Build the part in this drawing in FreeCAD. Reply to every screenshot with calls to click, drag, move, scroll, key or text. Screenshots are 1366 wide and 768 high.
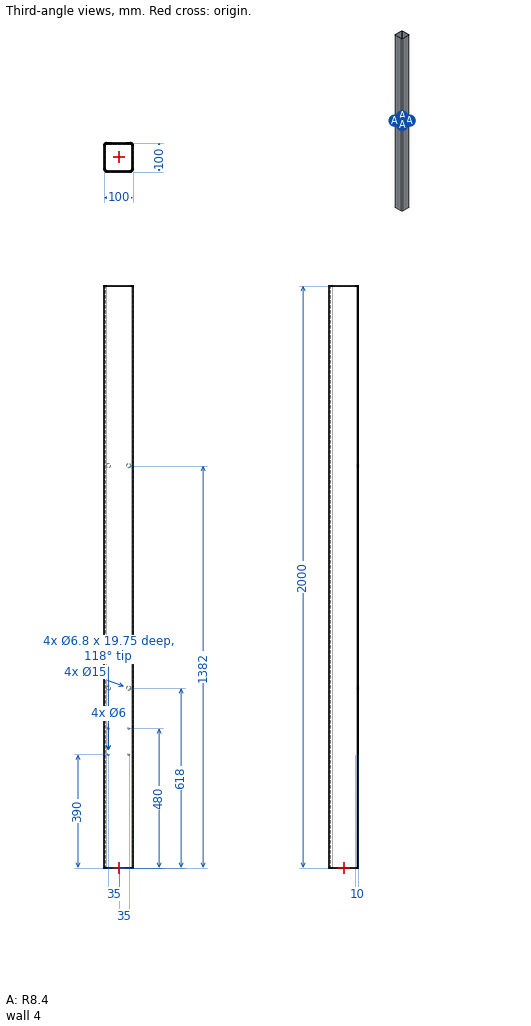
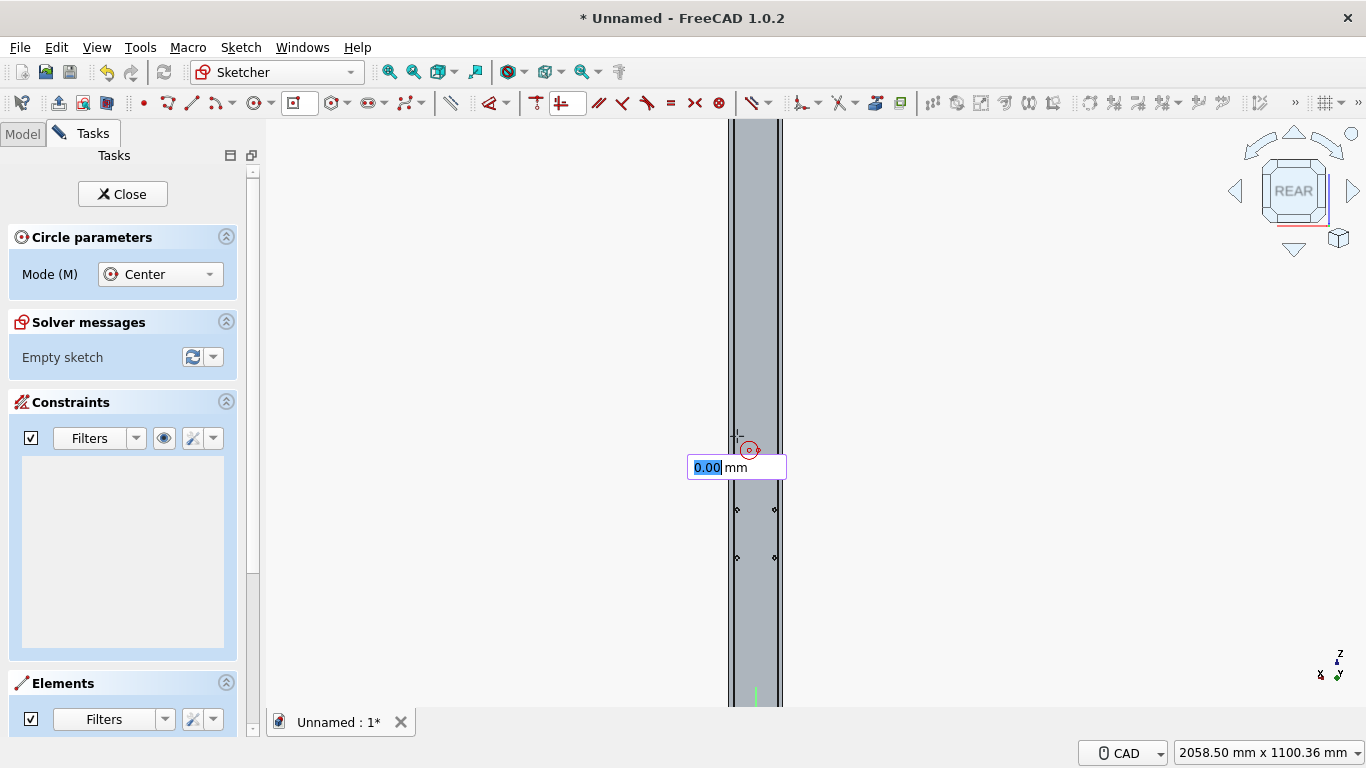
scroll(740, 433, up, 7)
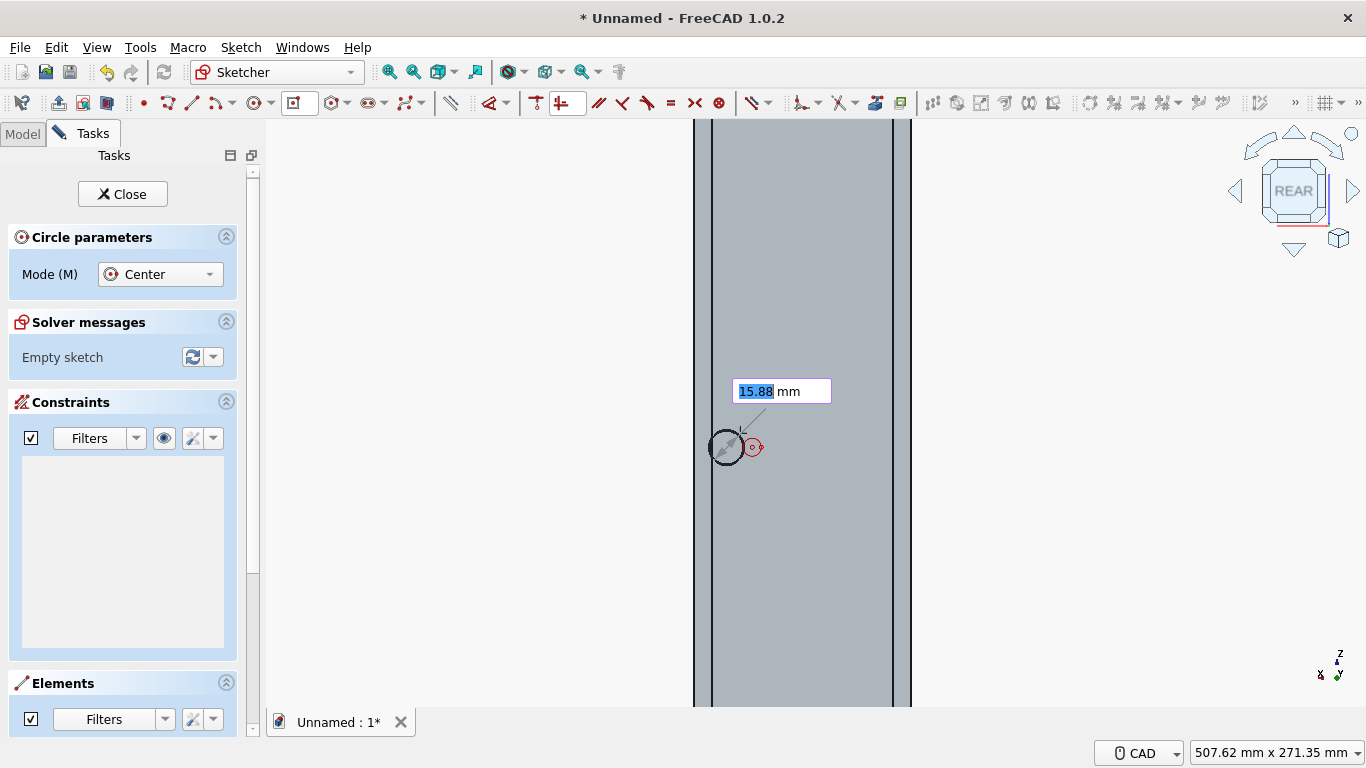
click(738, 432)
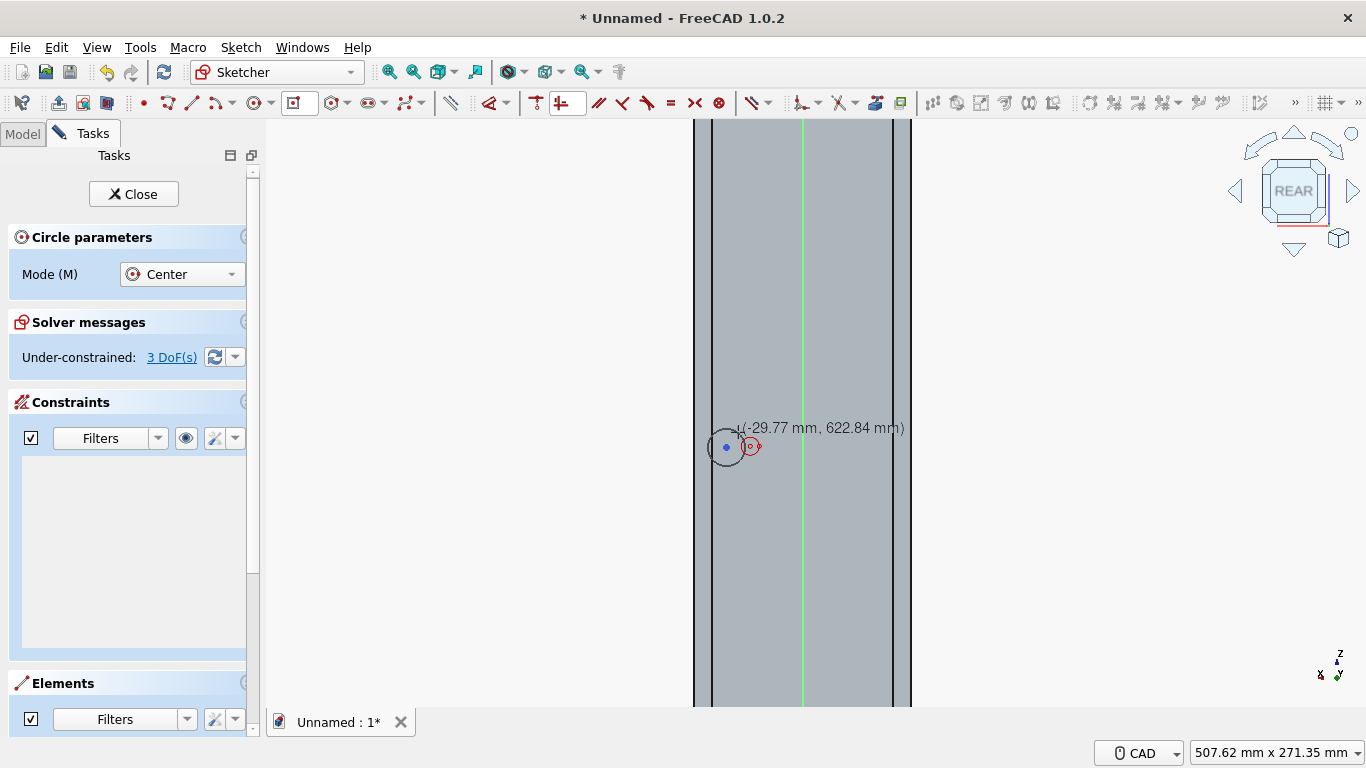
scroll(878, 443, up, 2)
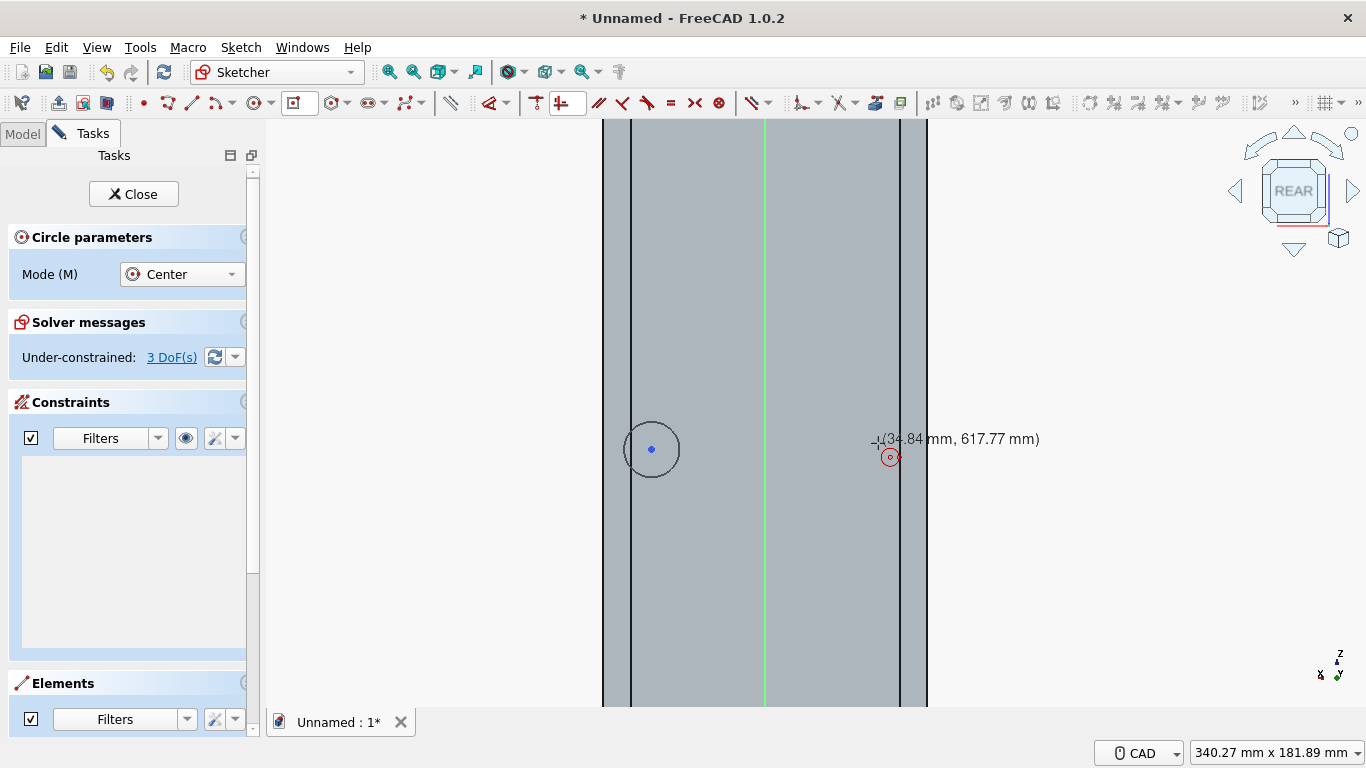
scroll(746, 435, down, 12)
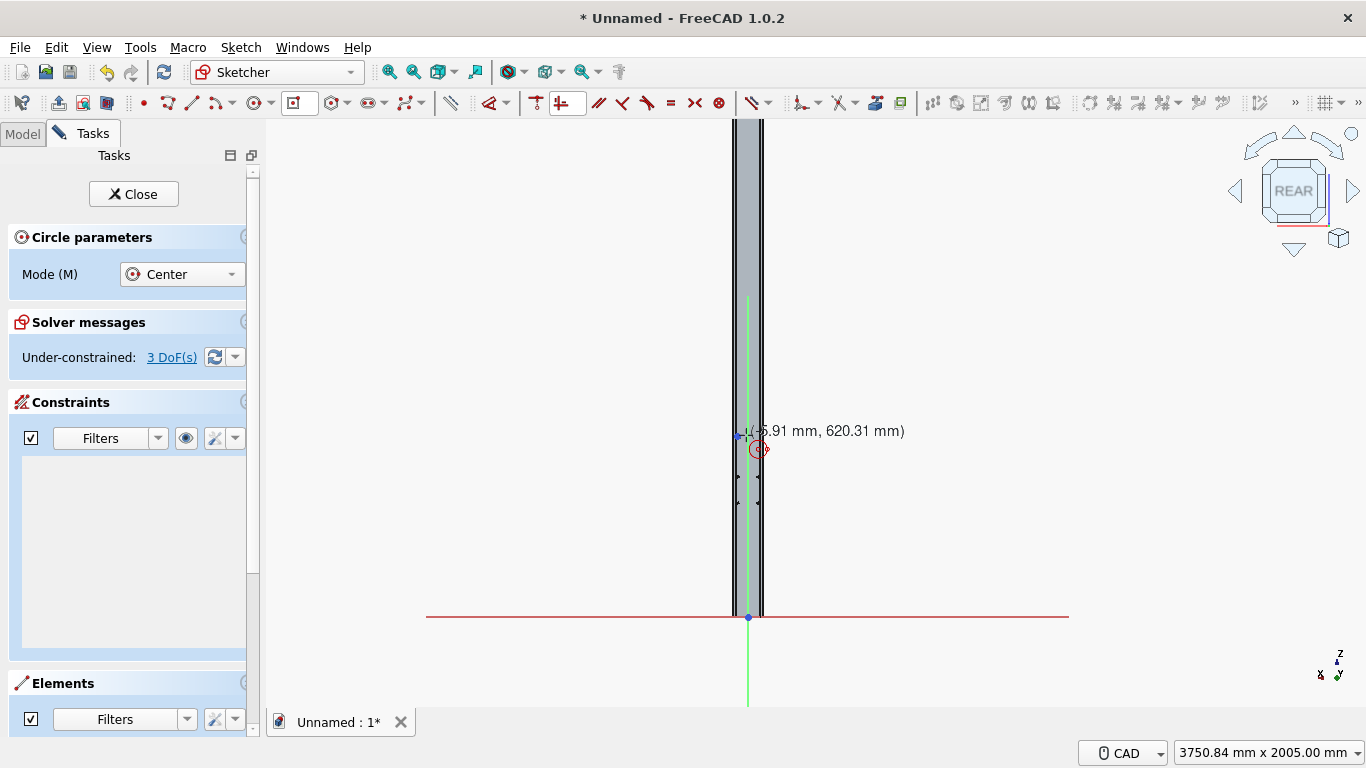
scroll(758, 436, up, 3)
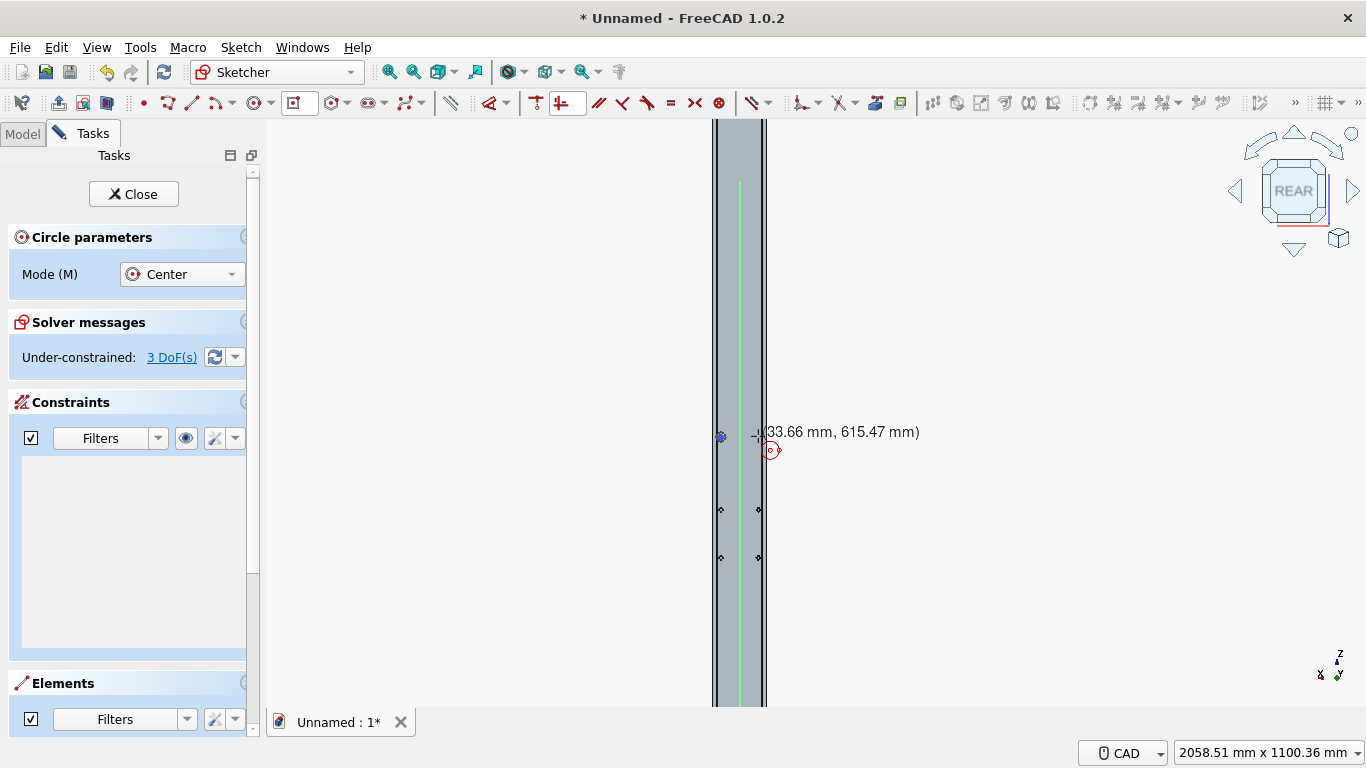
click(758, 436)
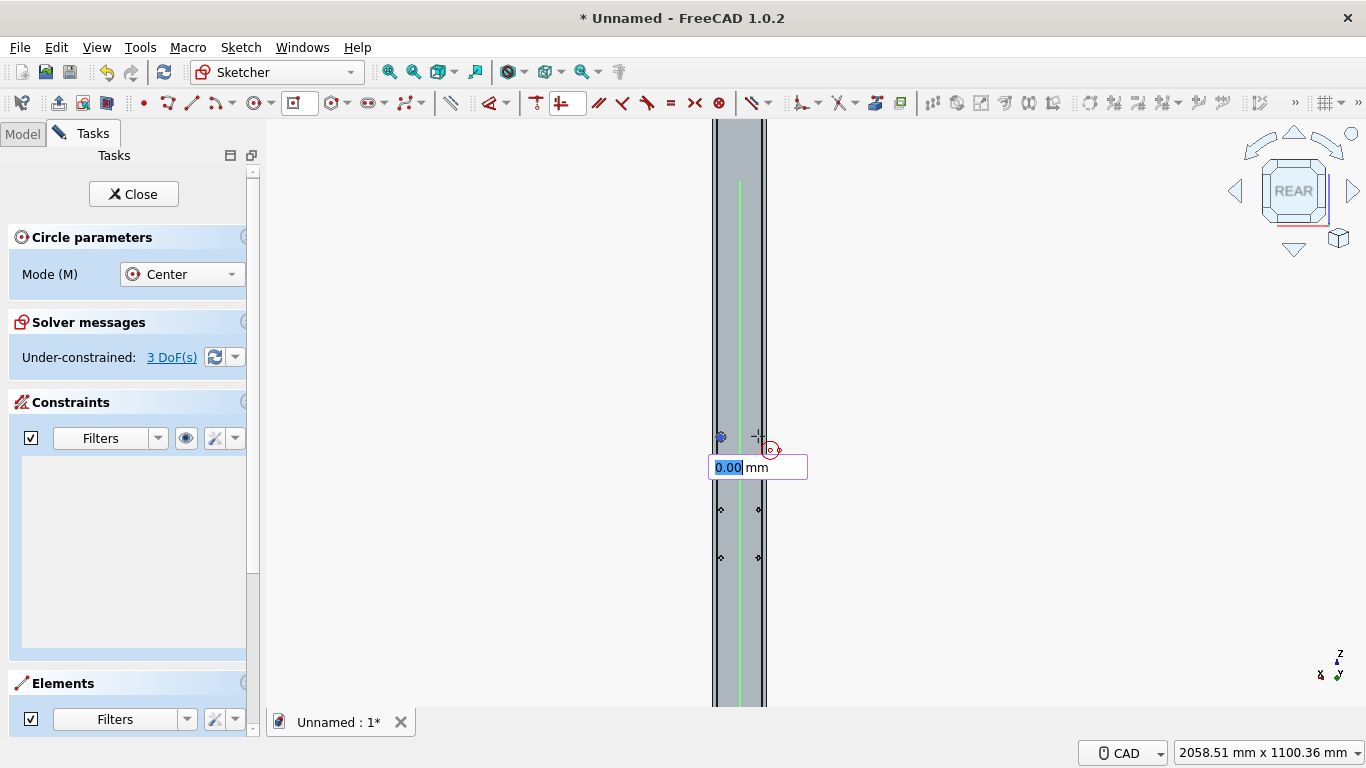
scroll(761, 433, up, 7)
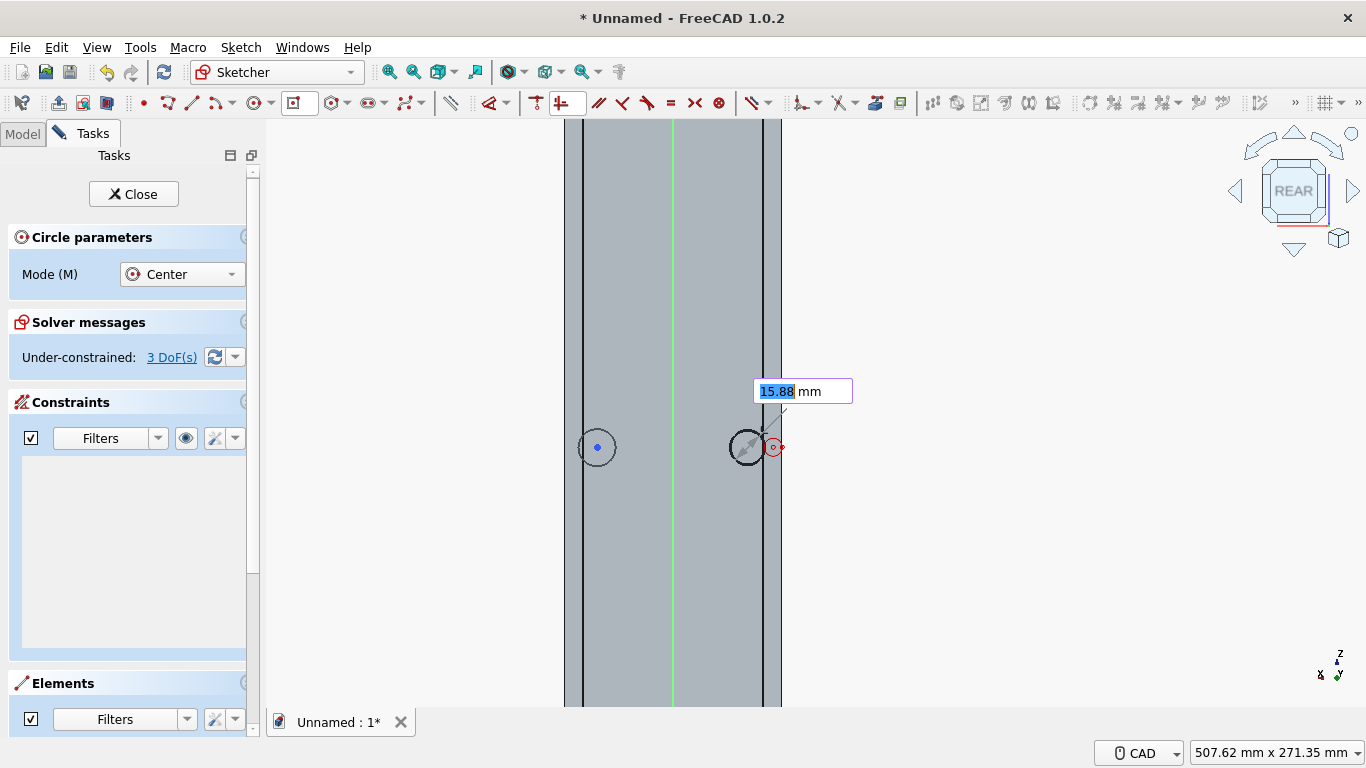
click(760, 432)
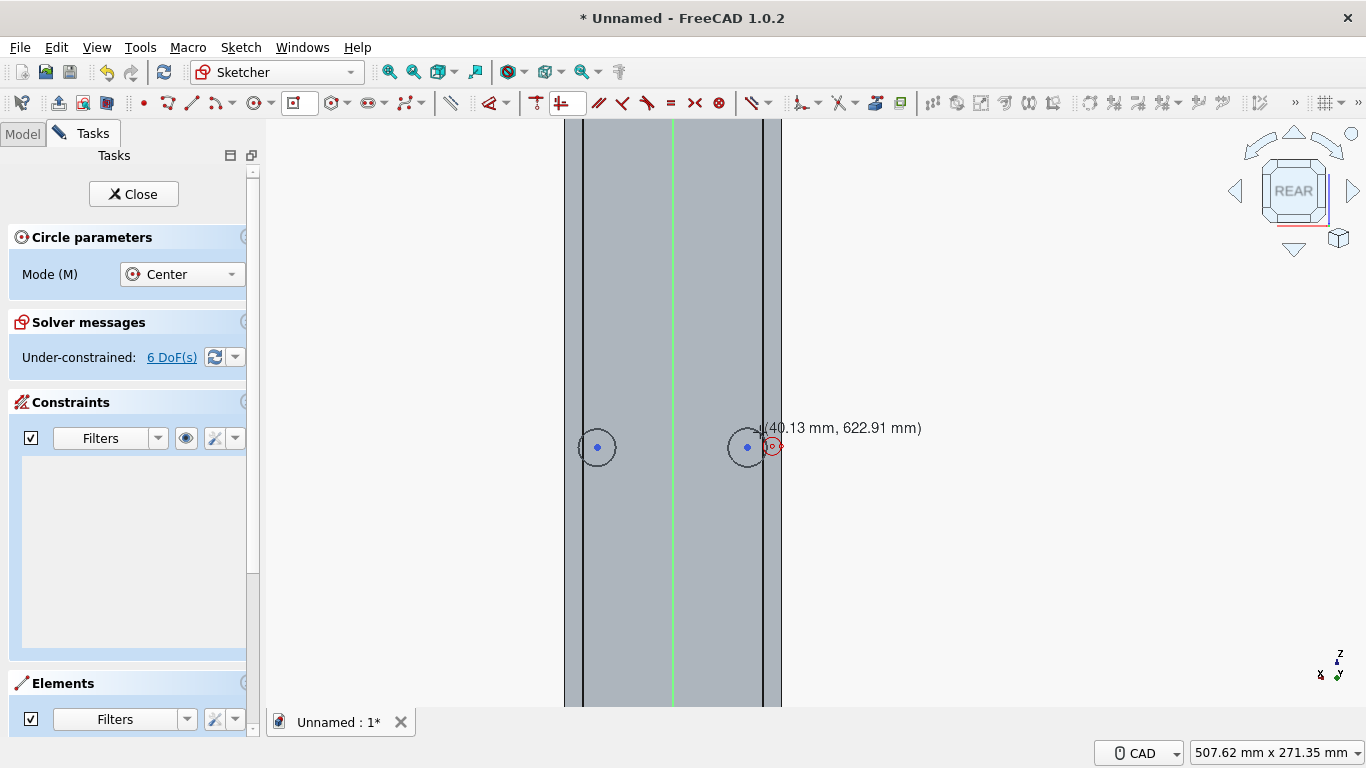
scroll(759, 434, down, 10)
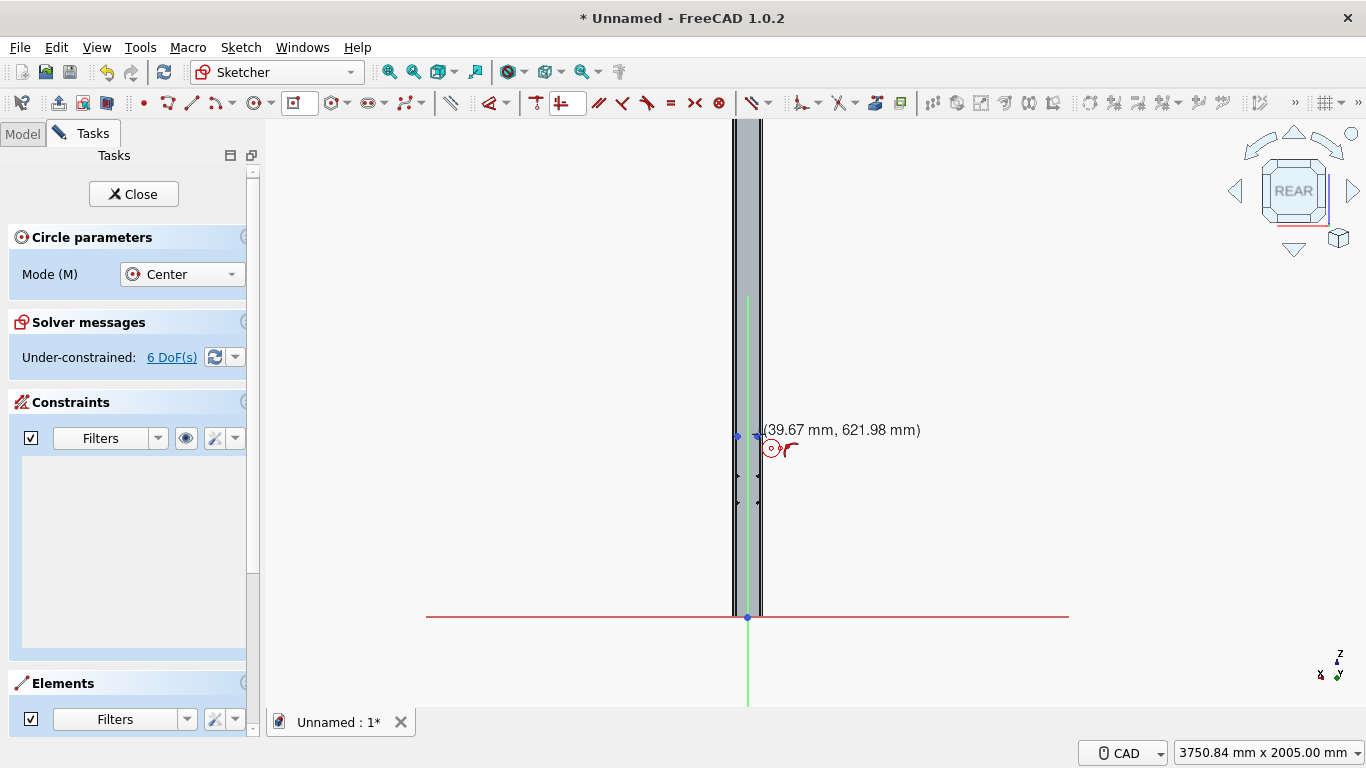
scroll(737, 212, up, 12)